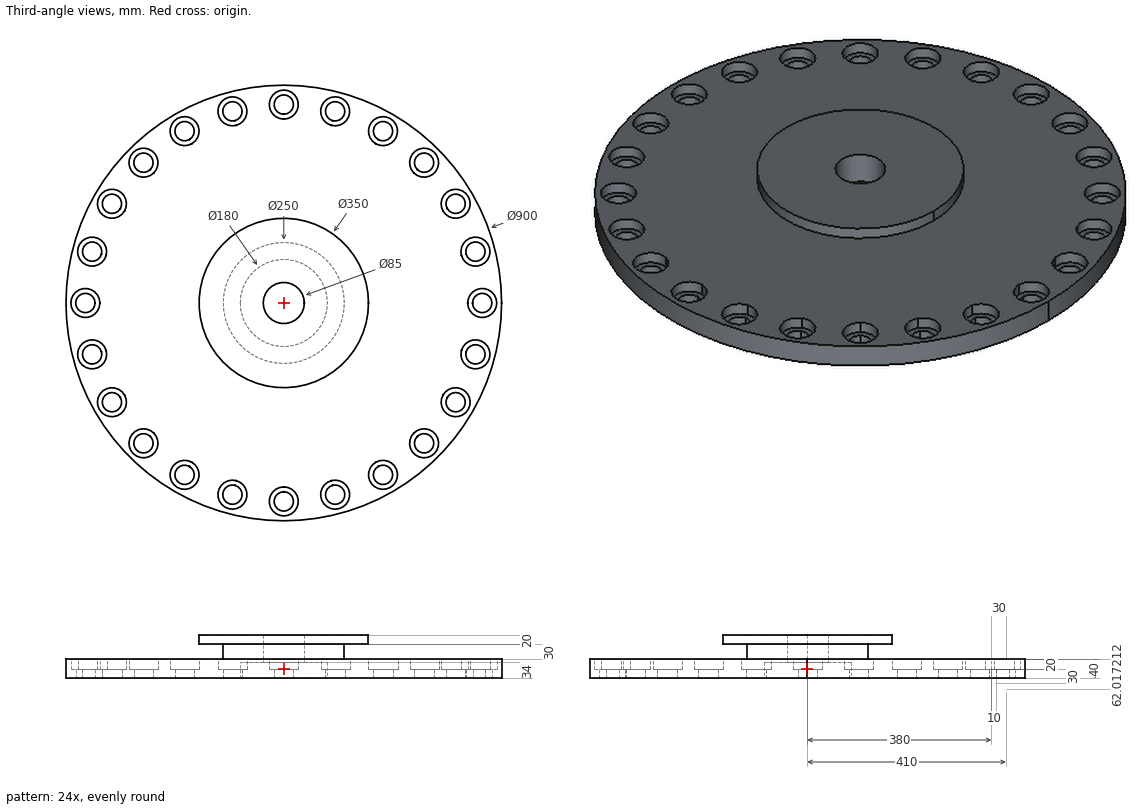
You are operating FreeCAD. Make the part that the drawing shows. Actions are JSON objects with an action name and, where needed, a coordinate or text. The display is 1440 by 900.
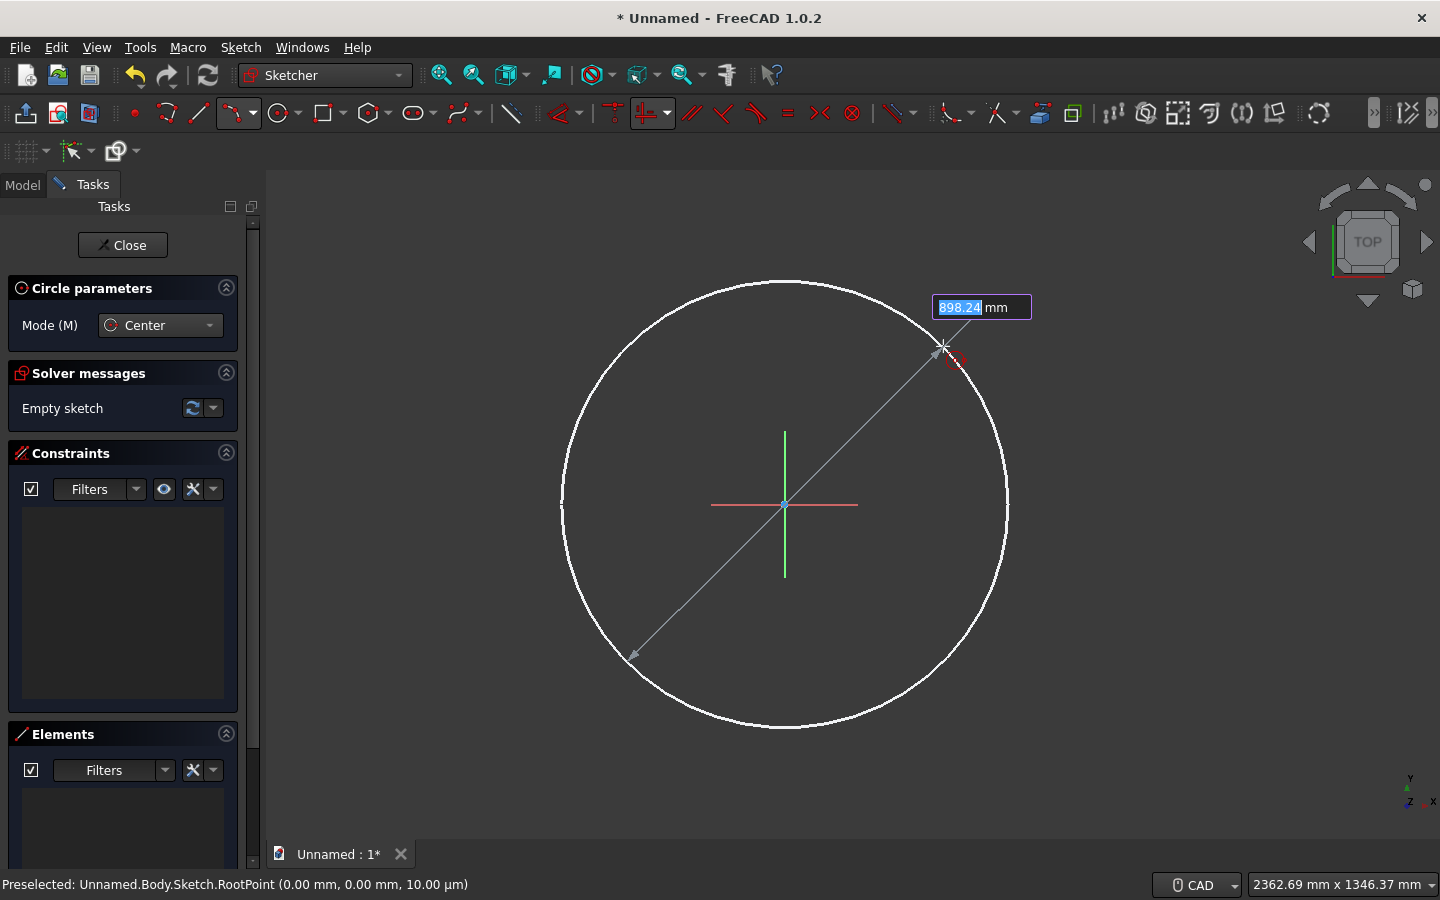
{"action": "type", "text": "900"}
{"action": "key", "text": "Return"}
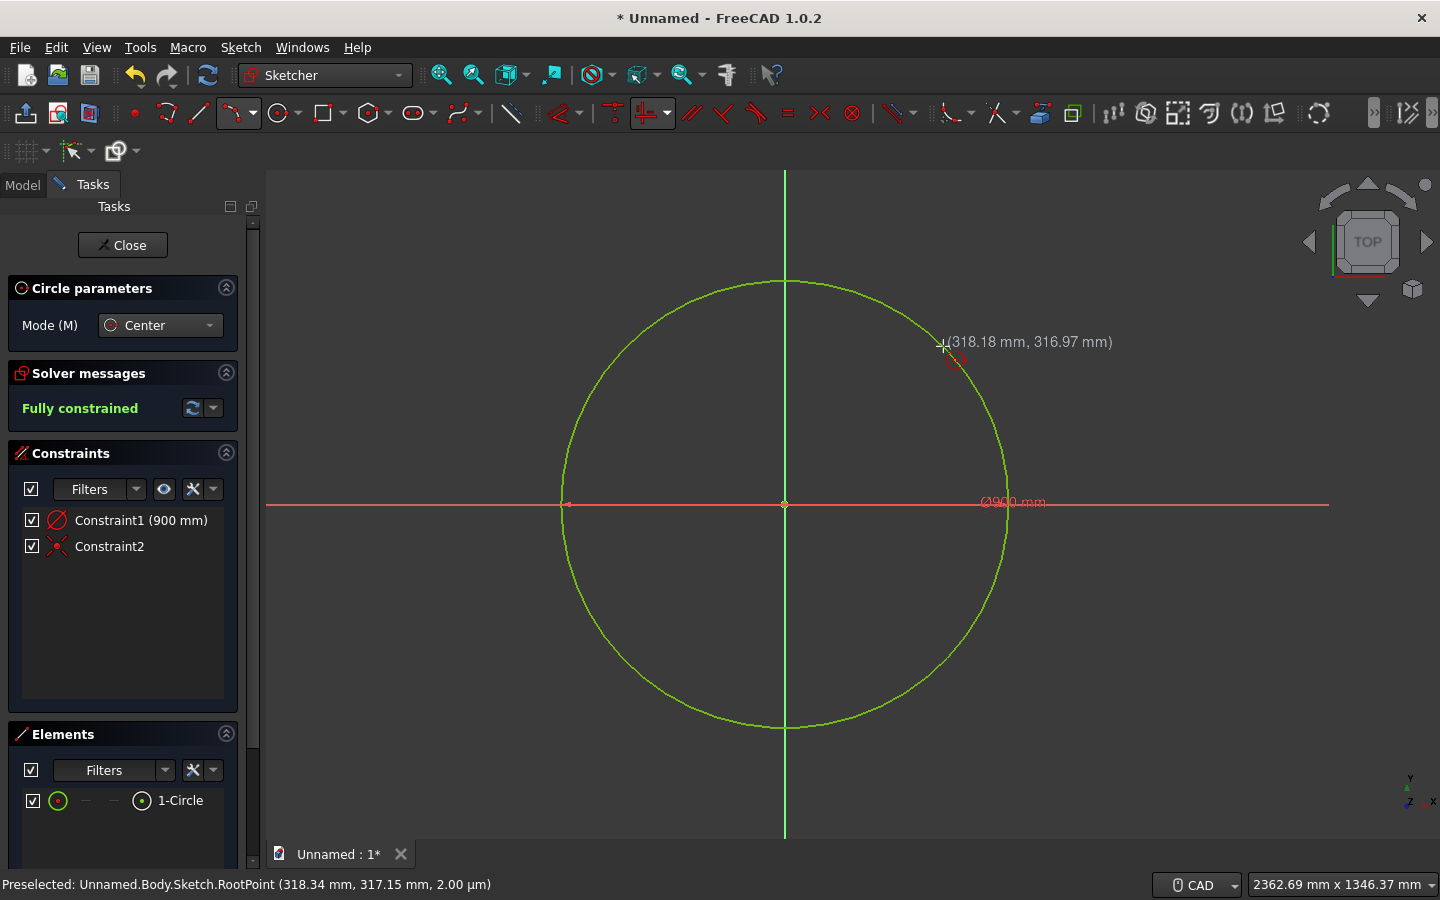
{"action": "left_click", "coordinate": [785, 504]}
{"action": "mouse_move", "coordinate": [800, 490]}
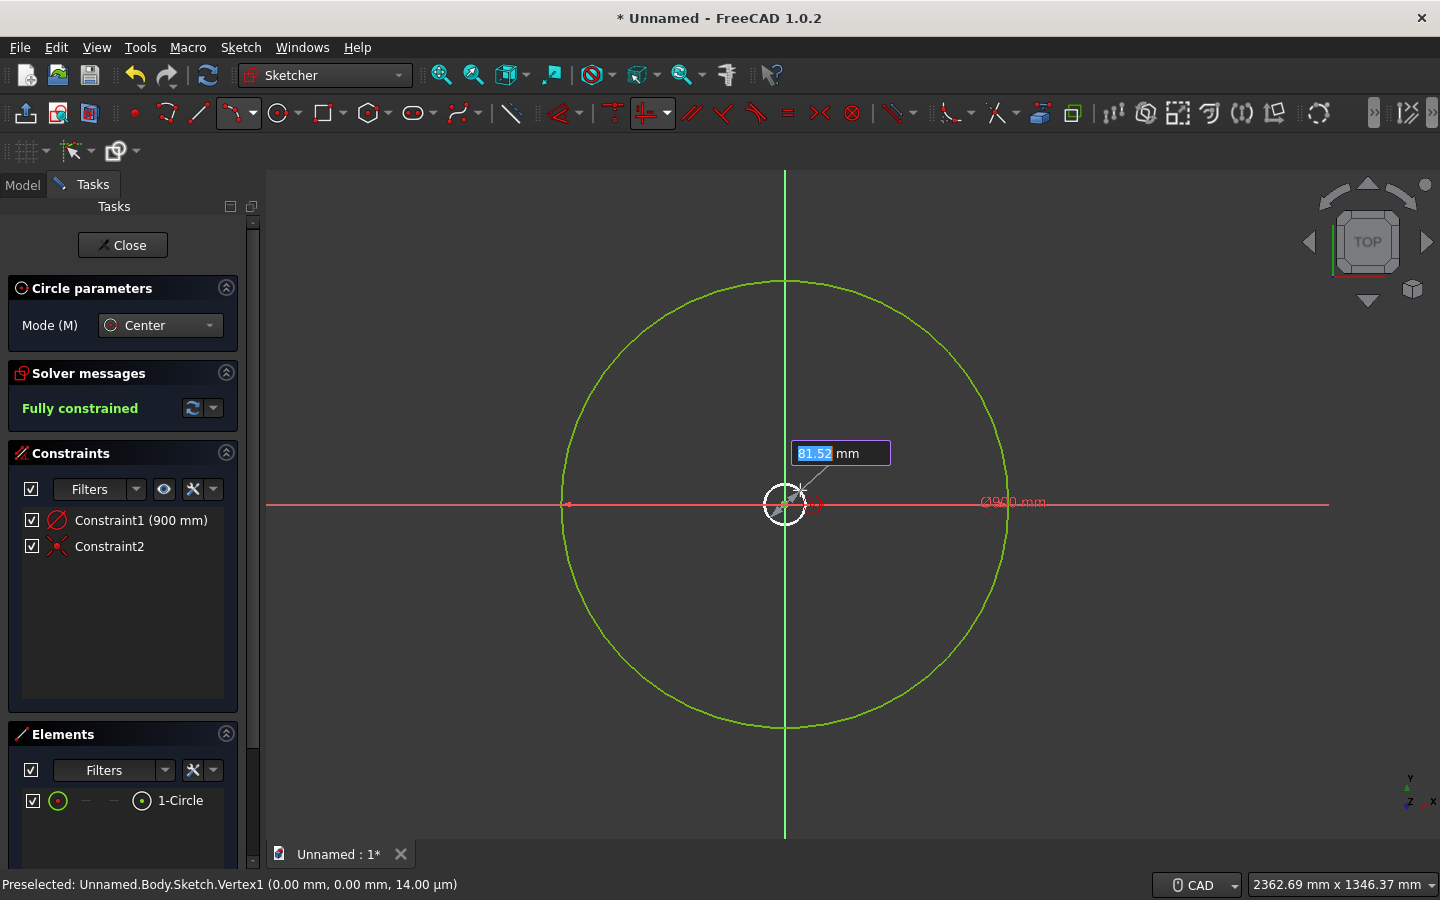
{"action": "type", "text": "85"}
{"action": "key", "text": "Return"}
{"action": "key", "text": "Escape"}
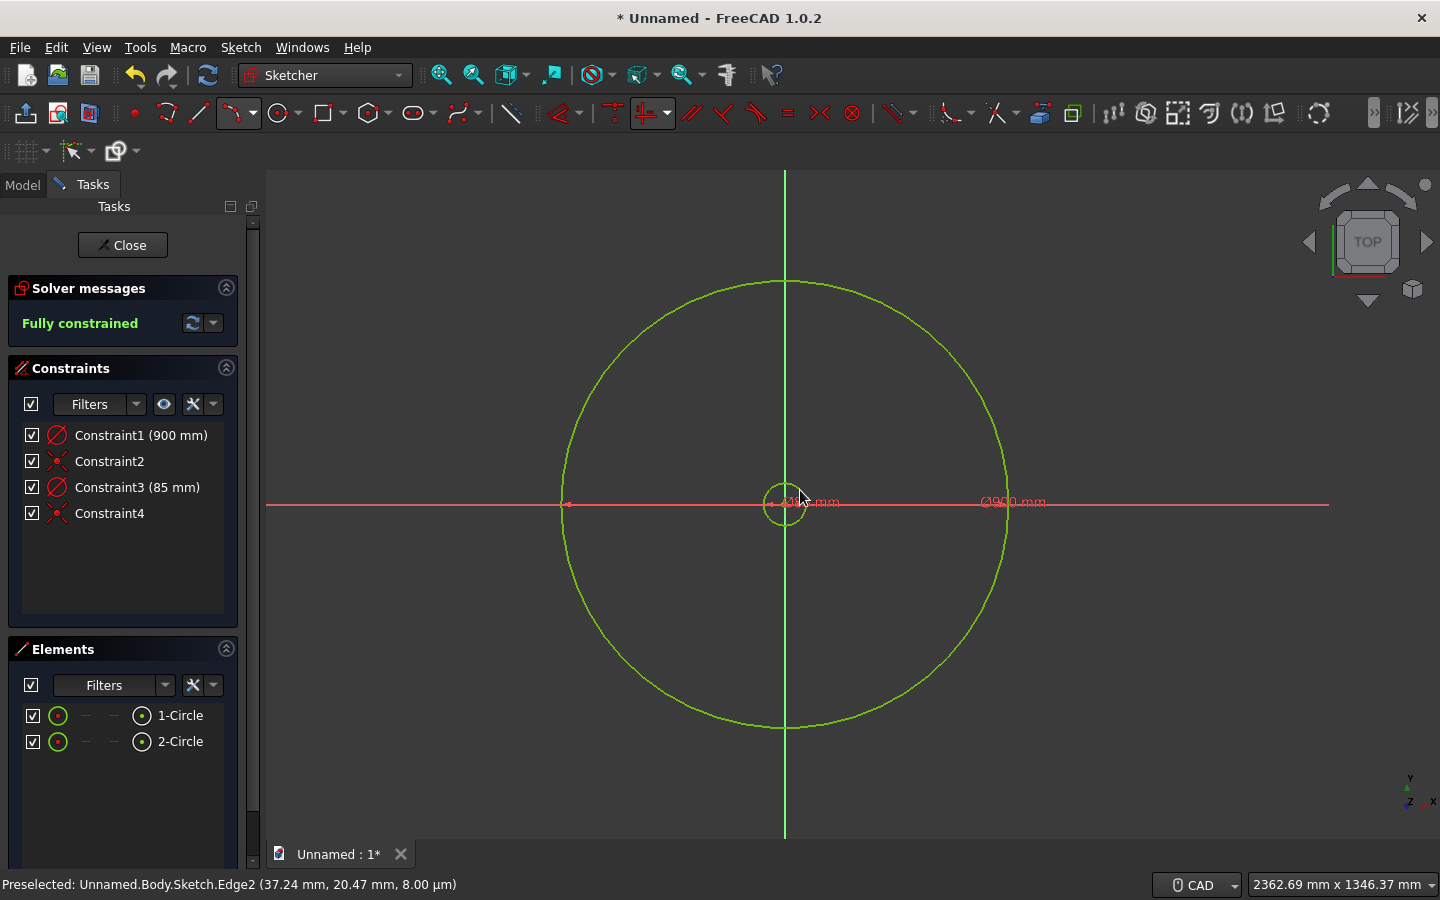
{"action": "left_click", "coordinate": [123, 245]}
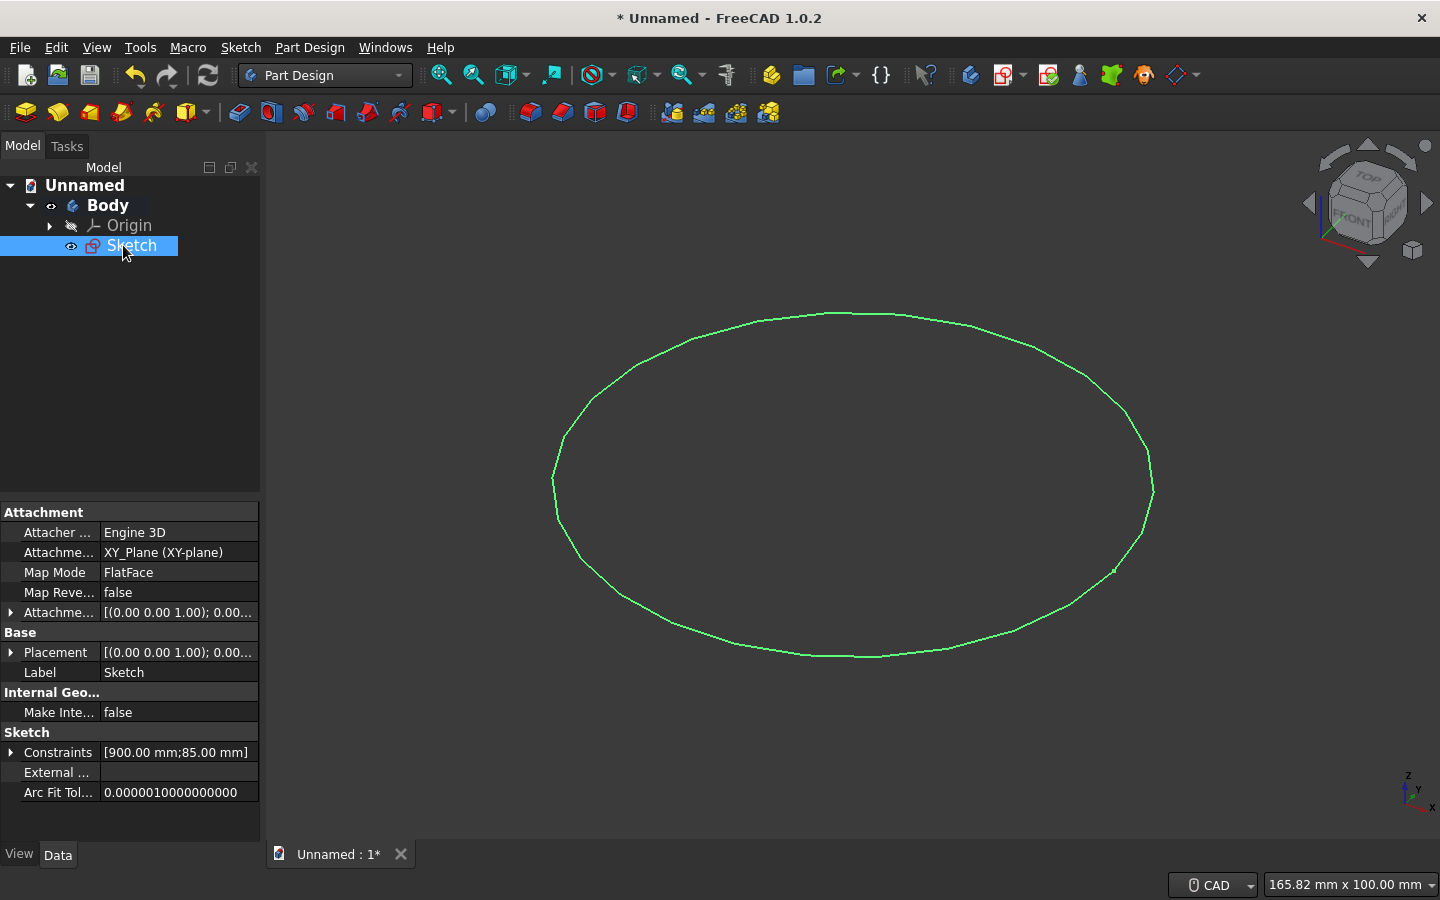
{"action": "left_click", "coordinate": [26, 112]}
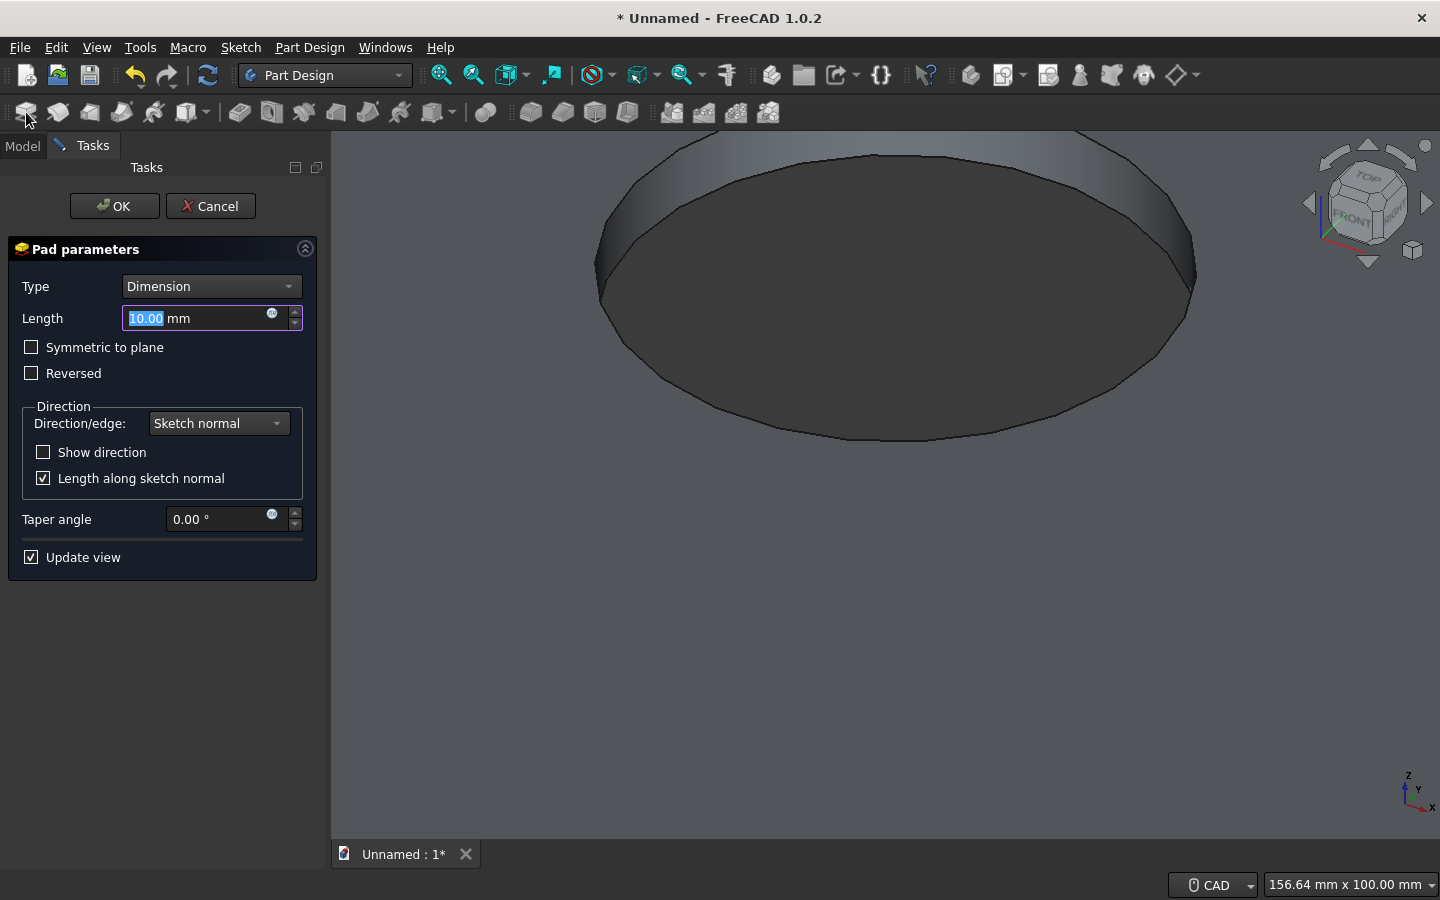
{"action": "type", "text": "40"}
{"action": "key", "text": "Tab"}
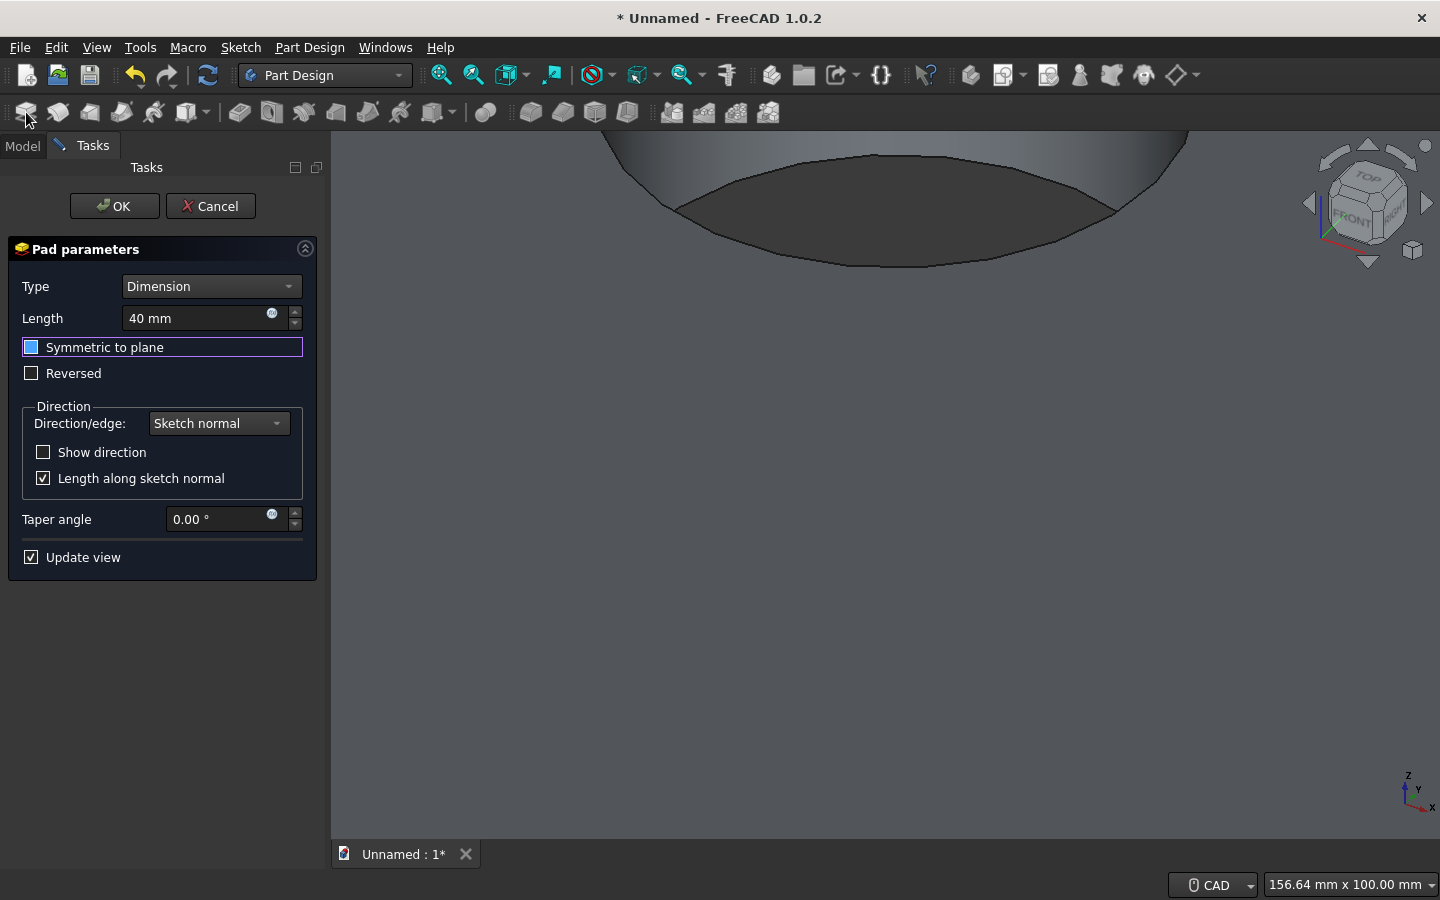
{"action": "left_click", "coordinate": [30, 347]}